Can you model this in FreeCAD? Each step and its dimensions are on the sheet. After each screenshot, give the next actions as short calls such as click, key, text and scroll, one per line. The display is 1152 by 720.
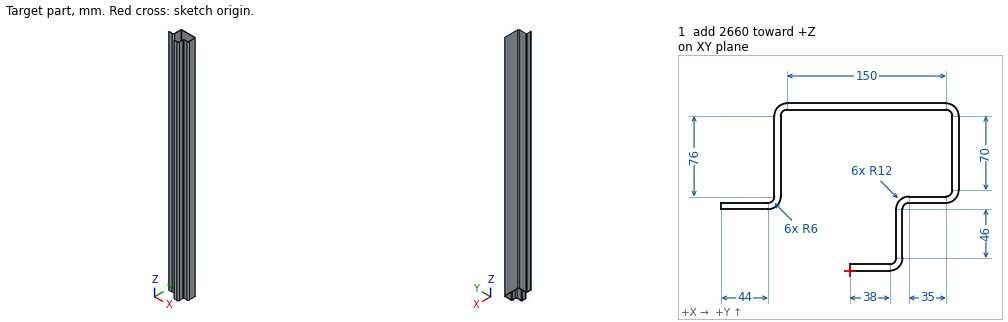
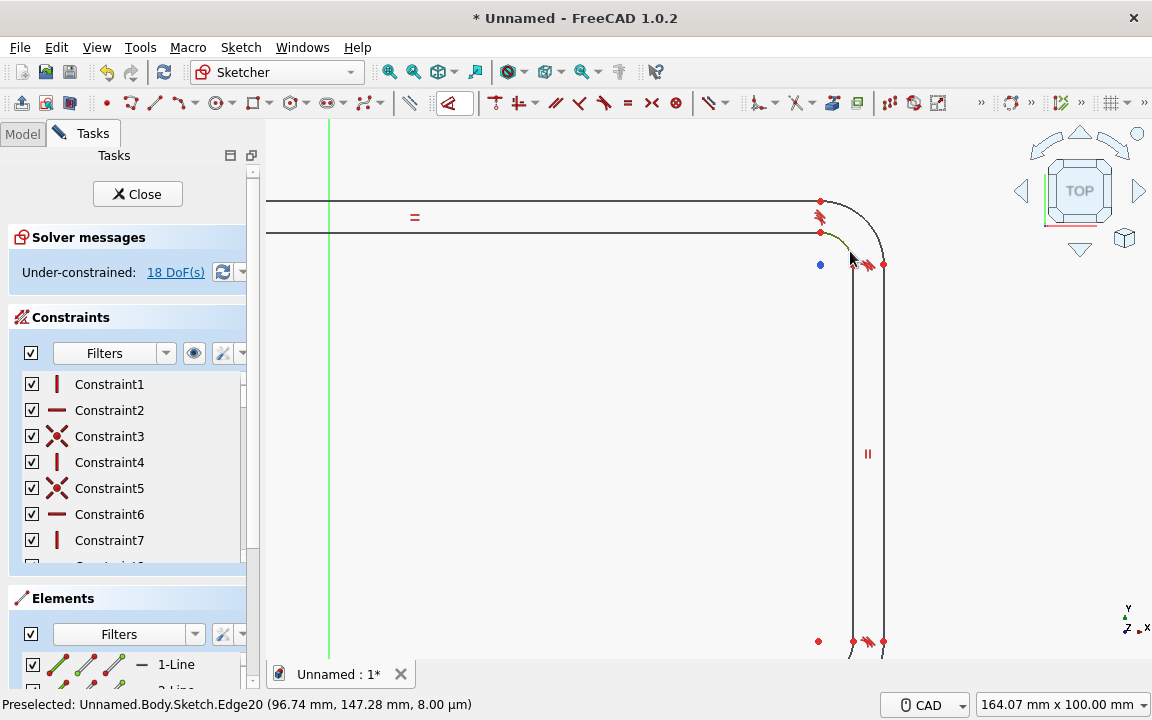
click(877, 236)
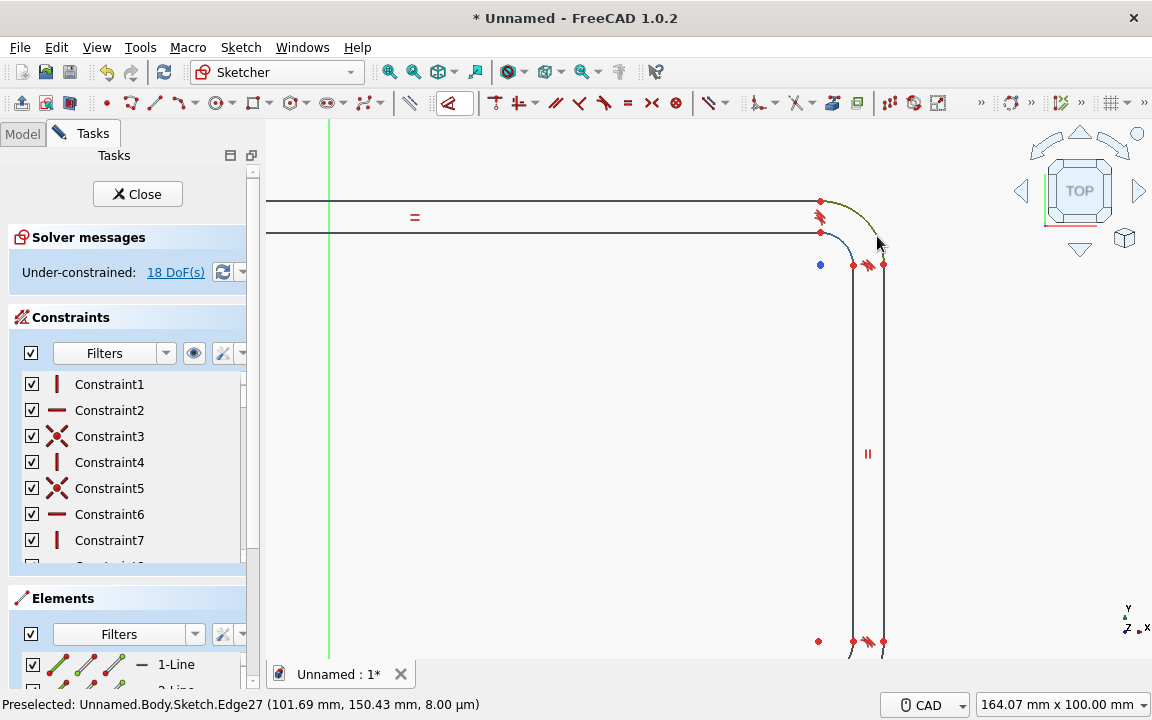
key(c)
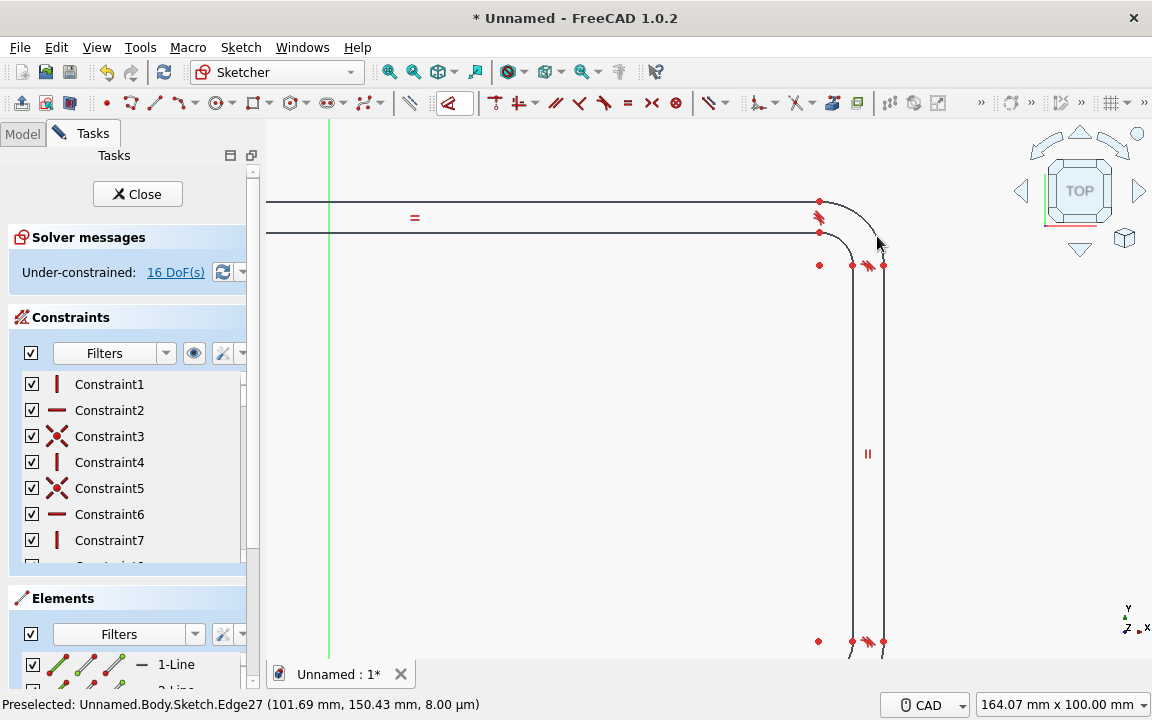
scroll(850, 251, down, 5)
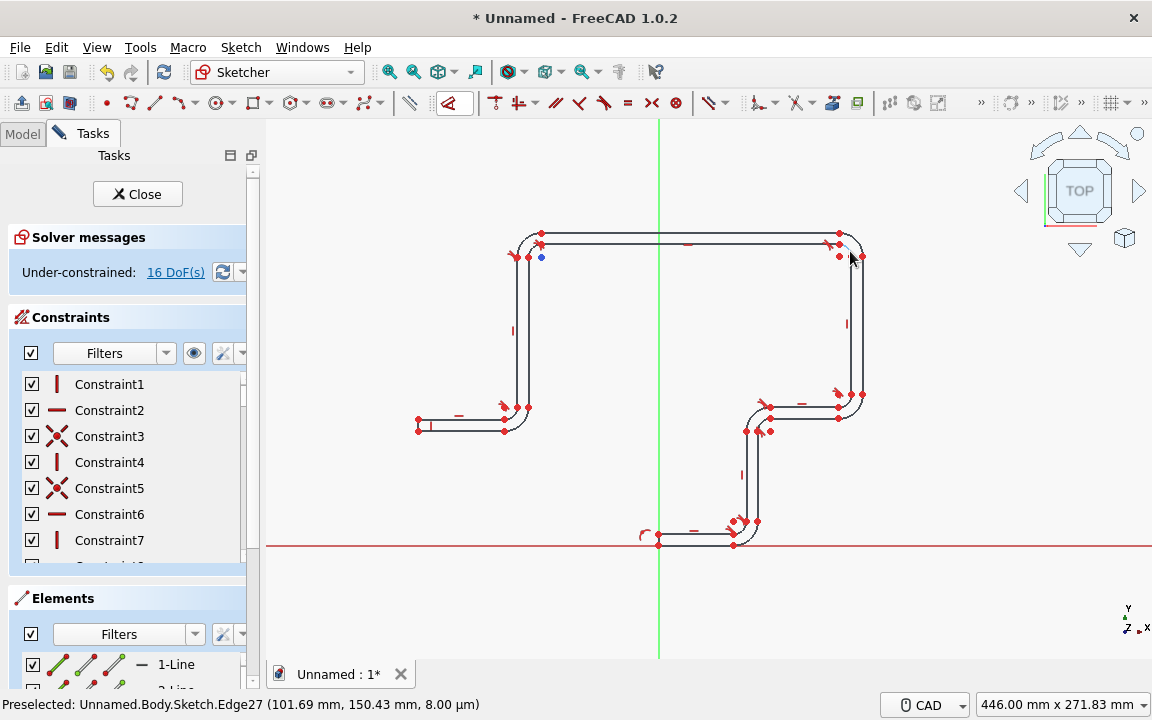
scroll(536, 246, up, 5)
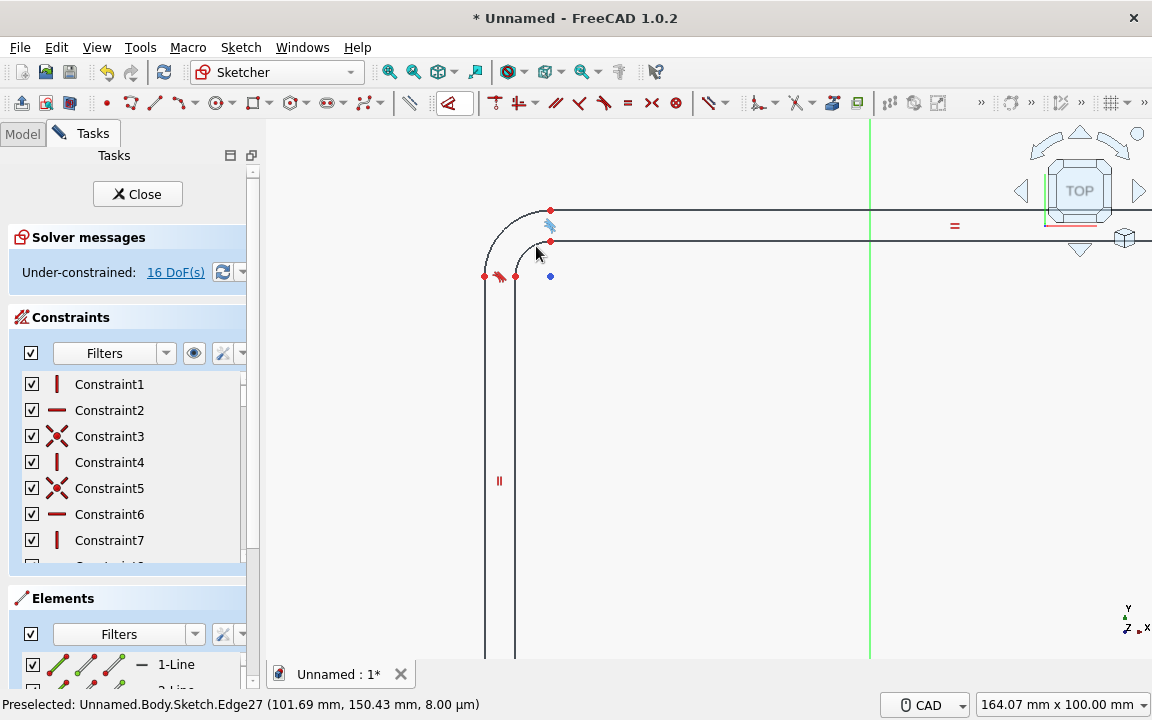
click(535, 245)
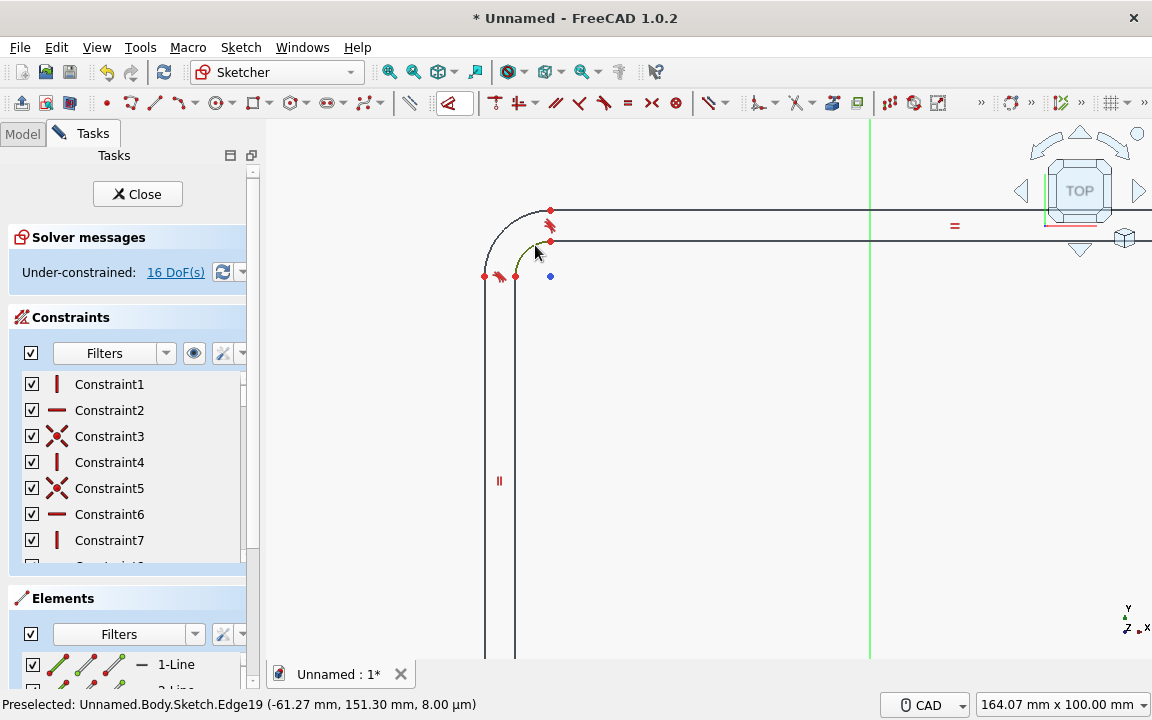
click(521, 218)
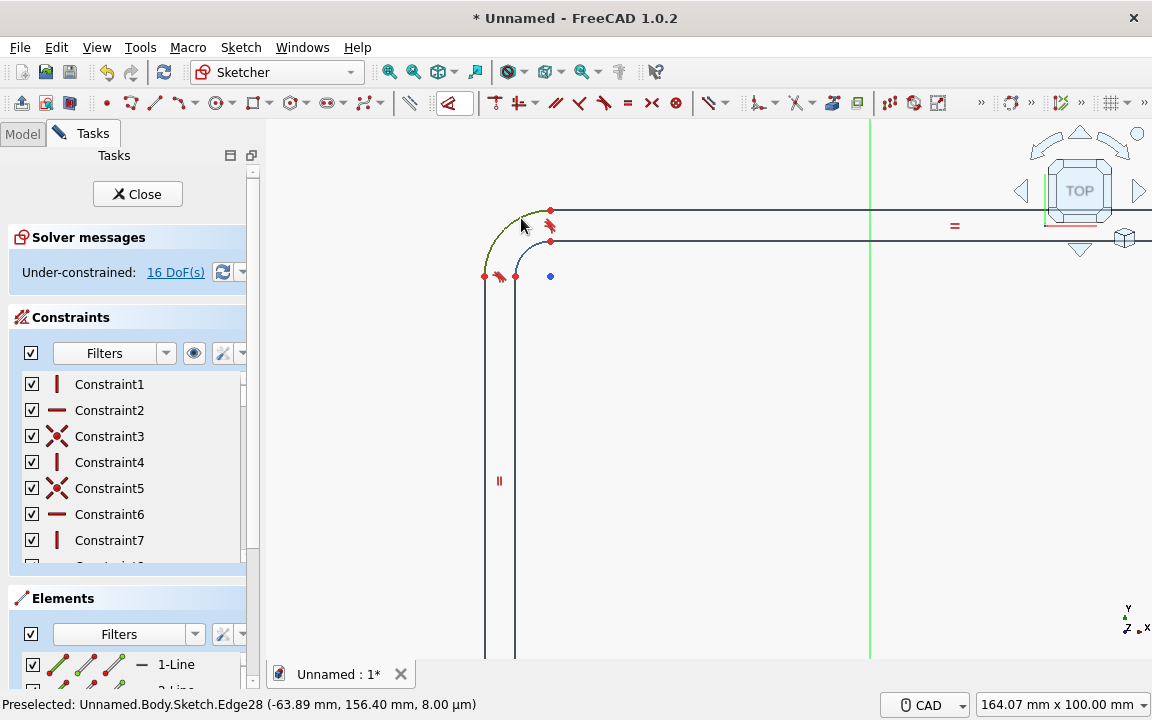
key(c)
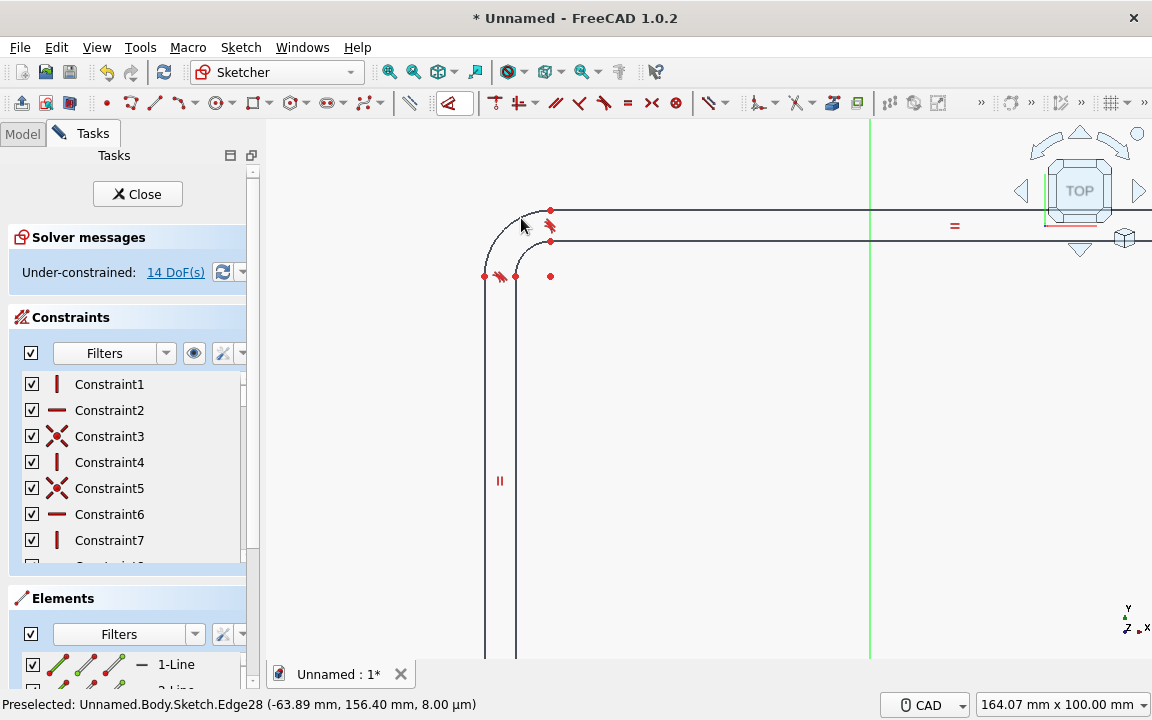
scroll(535, 246, down, 5)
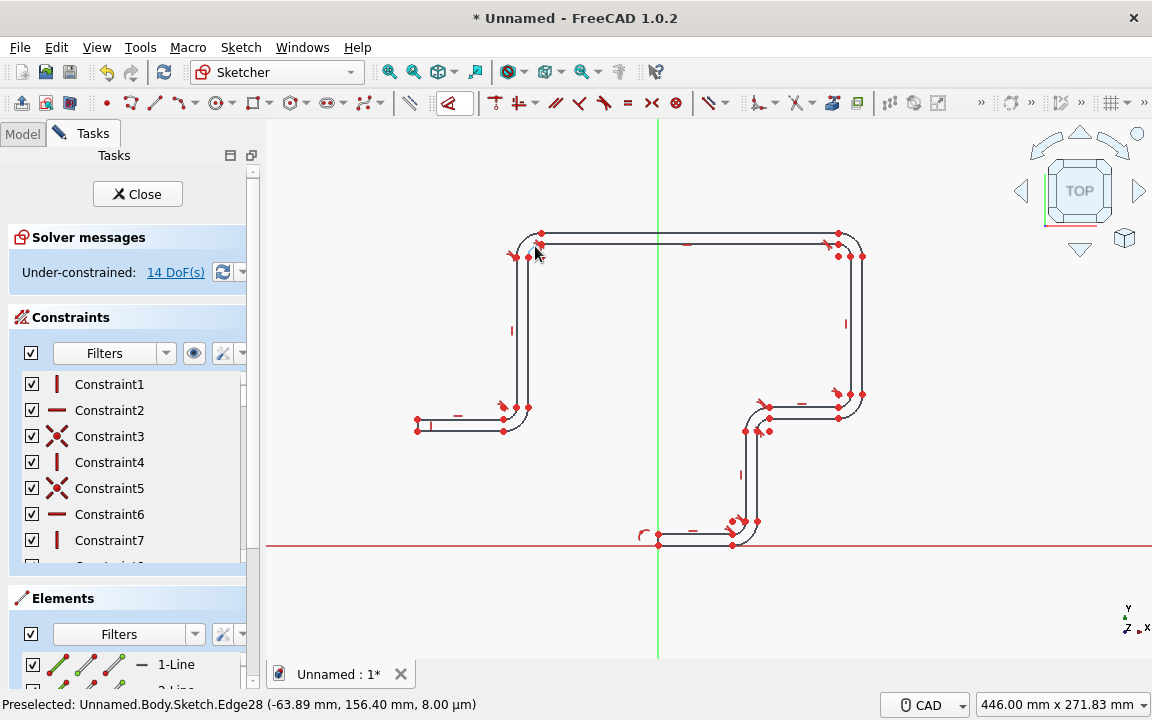
scroll(510, 419, up, 5)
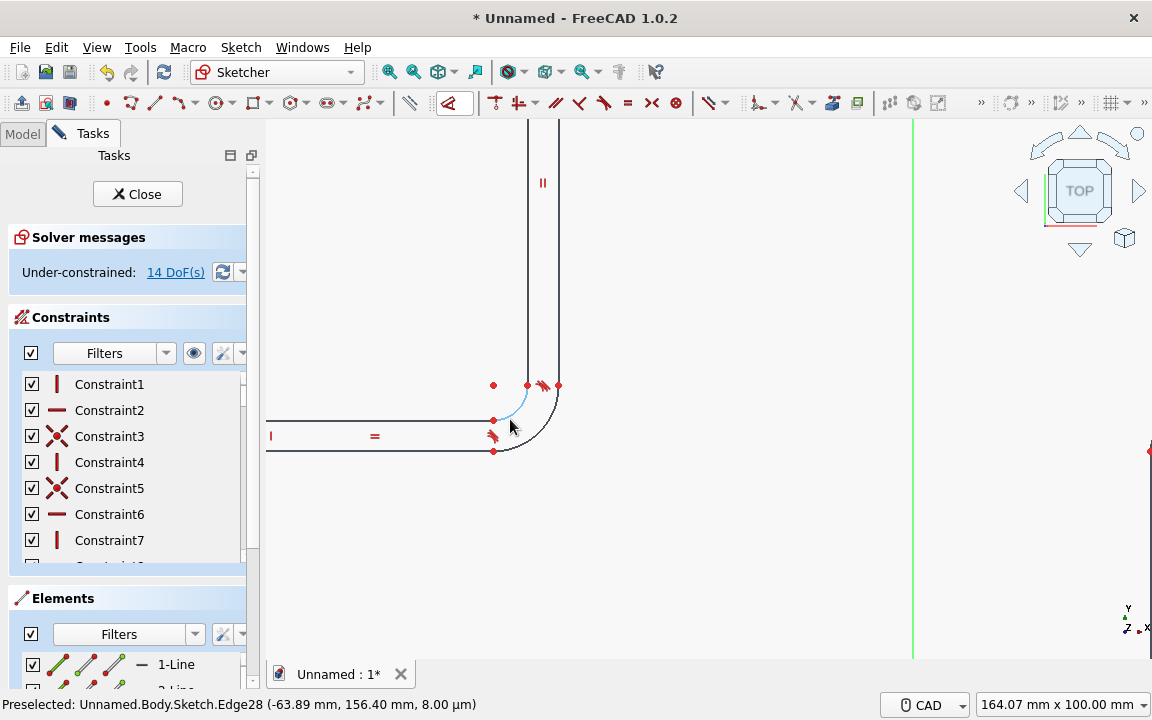
click(509, 417)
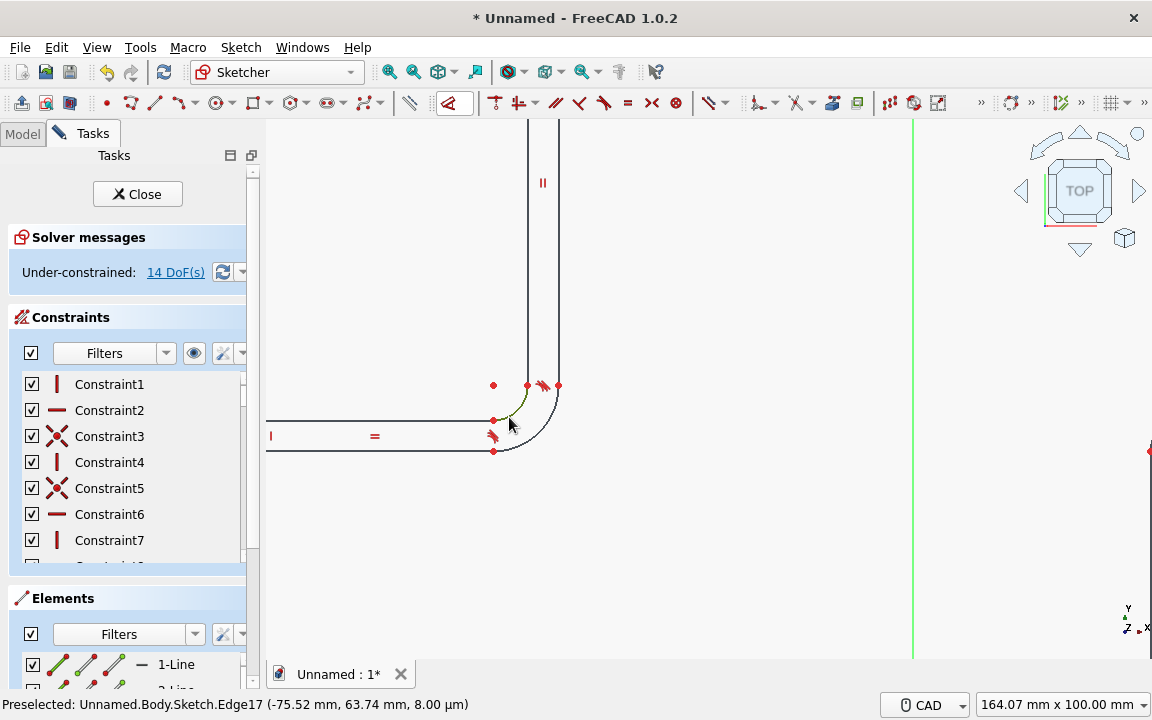
scroll(510, 420, down, 5)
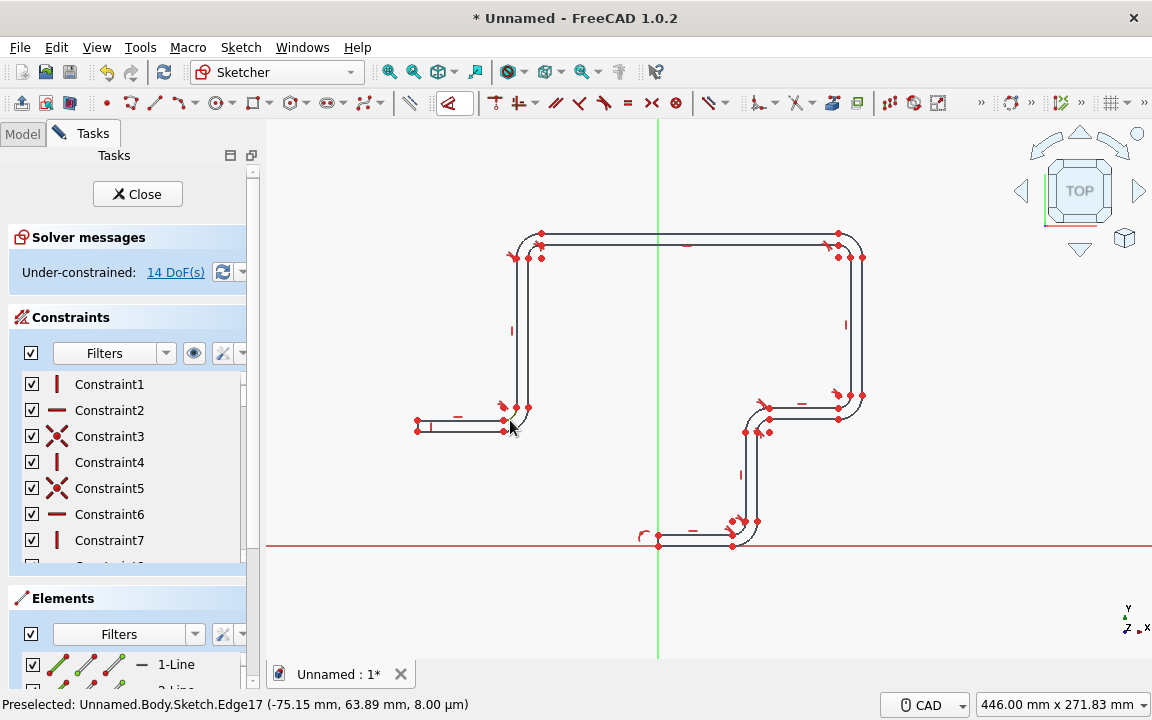
scroll(535, 247, up, 5)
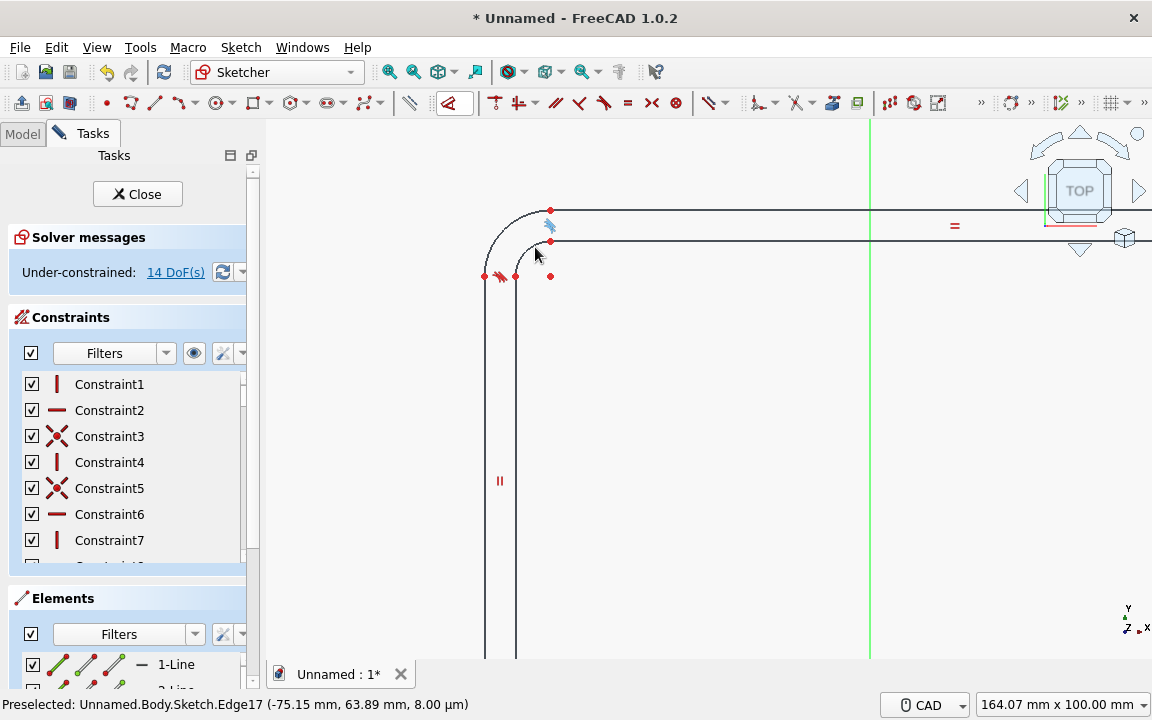
click(535, 245)